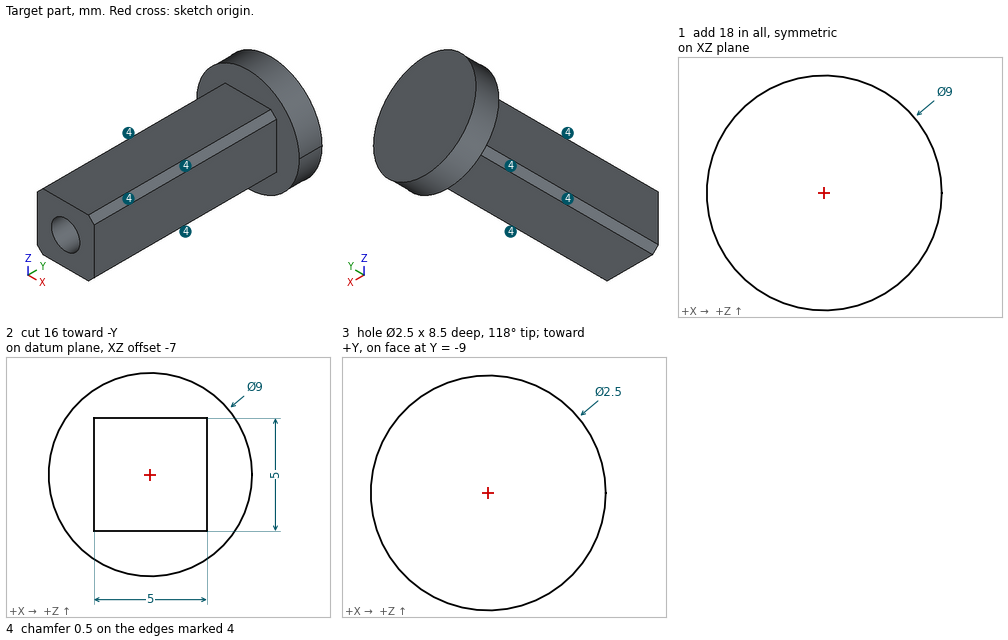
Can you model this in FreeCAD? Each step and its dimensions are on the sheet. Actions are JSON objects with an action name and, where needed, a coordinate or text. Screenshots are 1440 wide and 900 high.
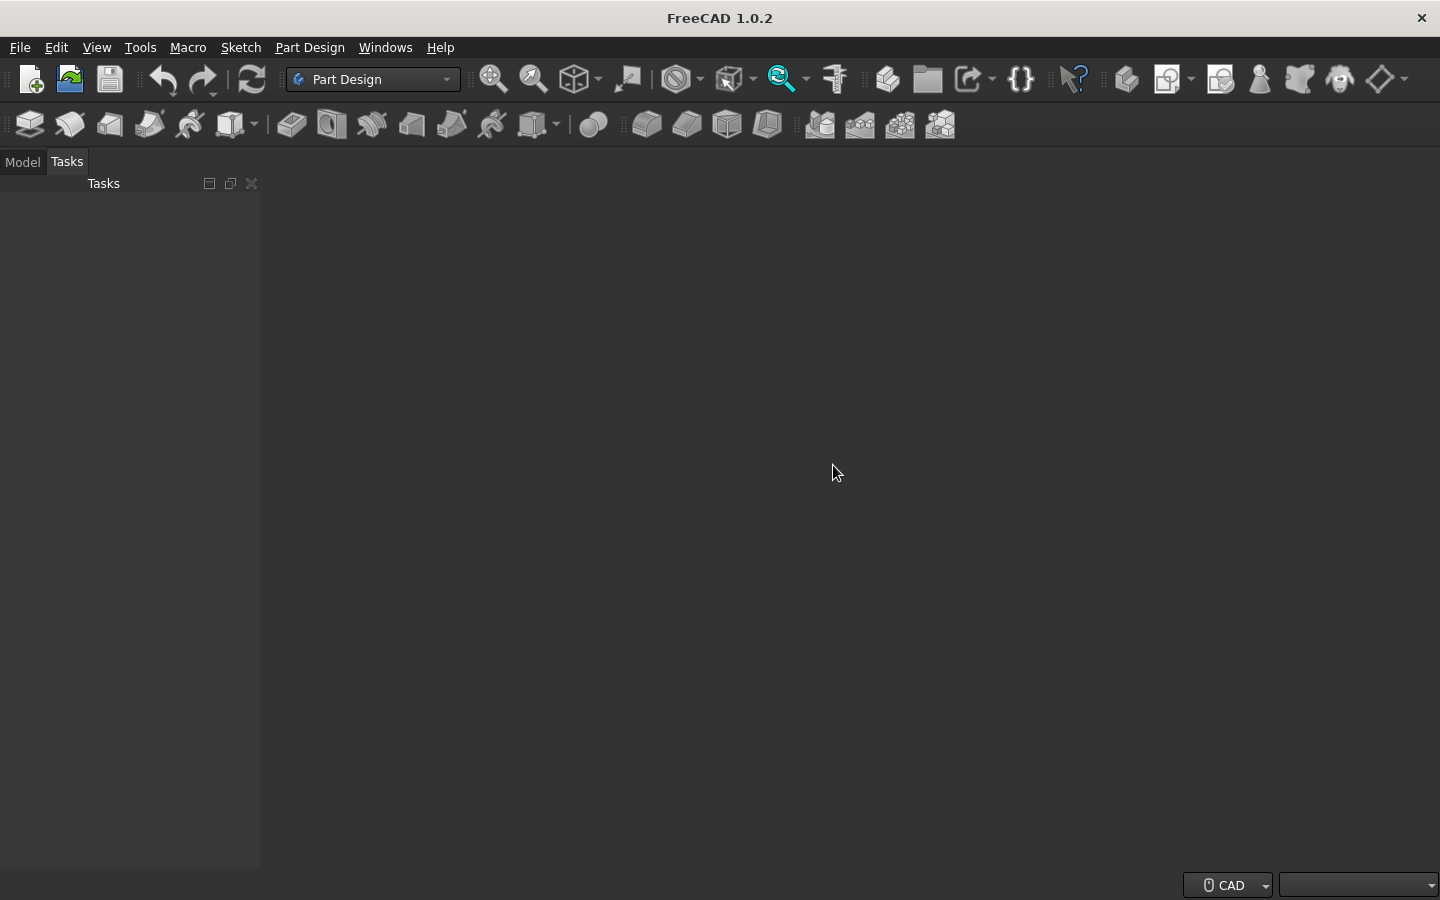
{"action": "left_click", "coordinate": [30, 80]}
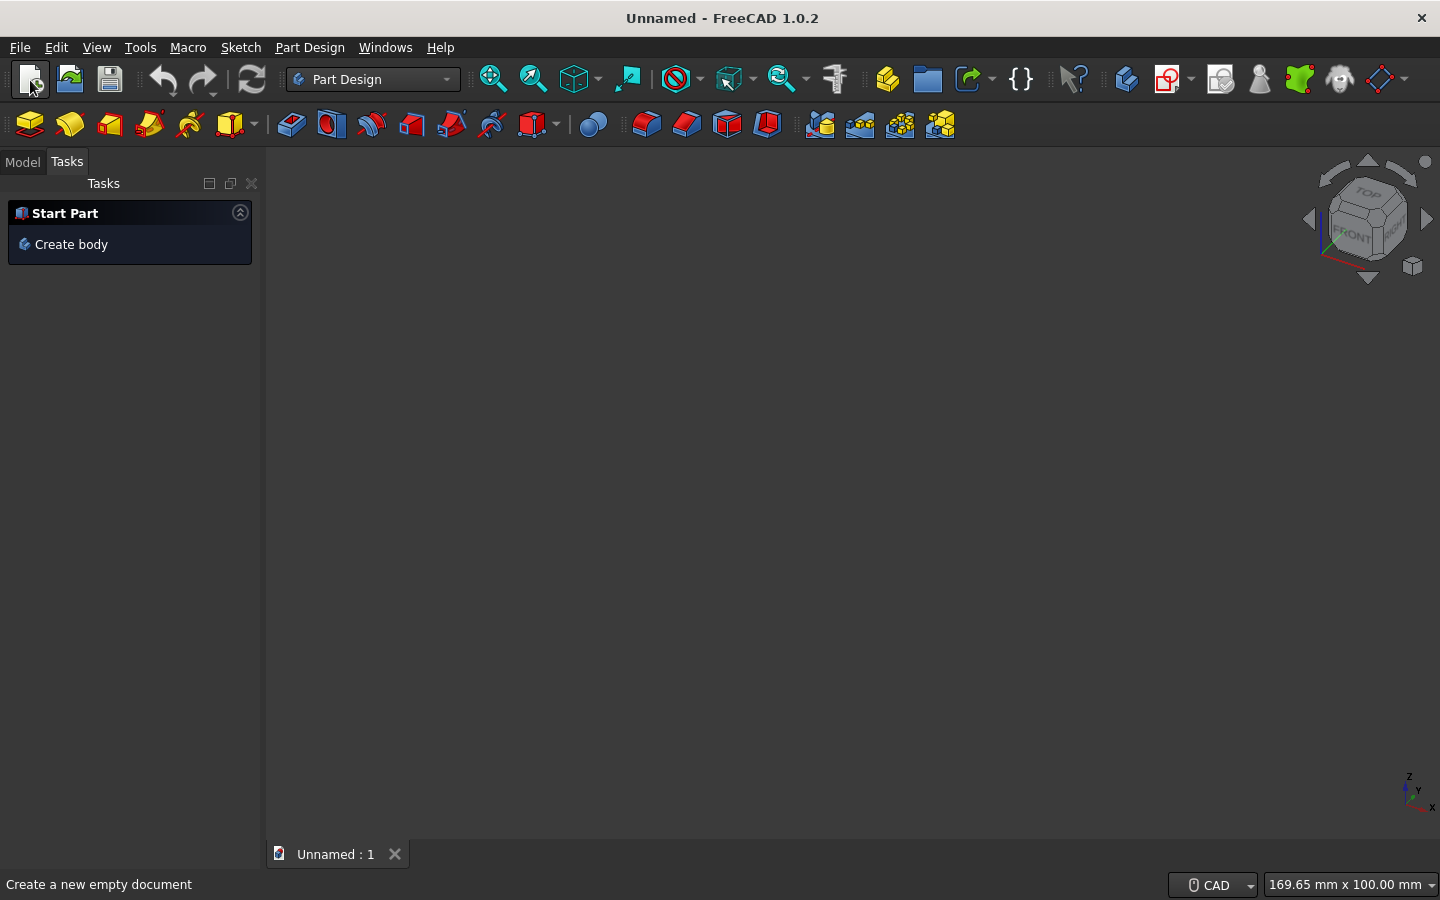
{"action": "left_click", "coordinate": [1168, 80]}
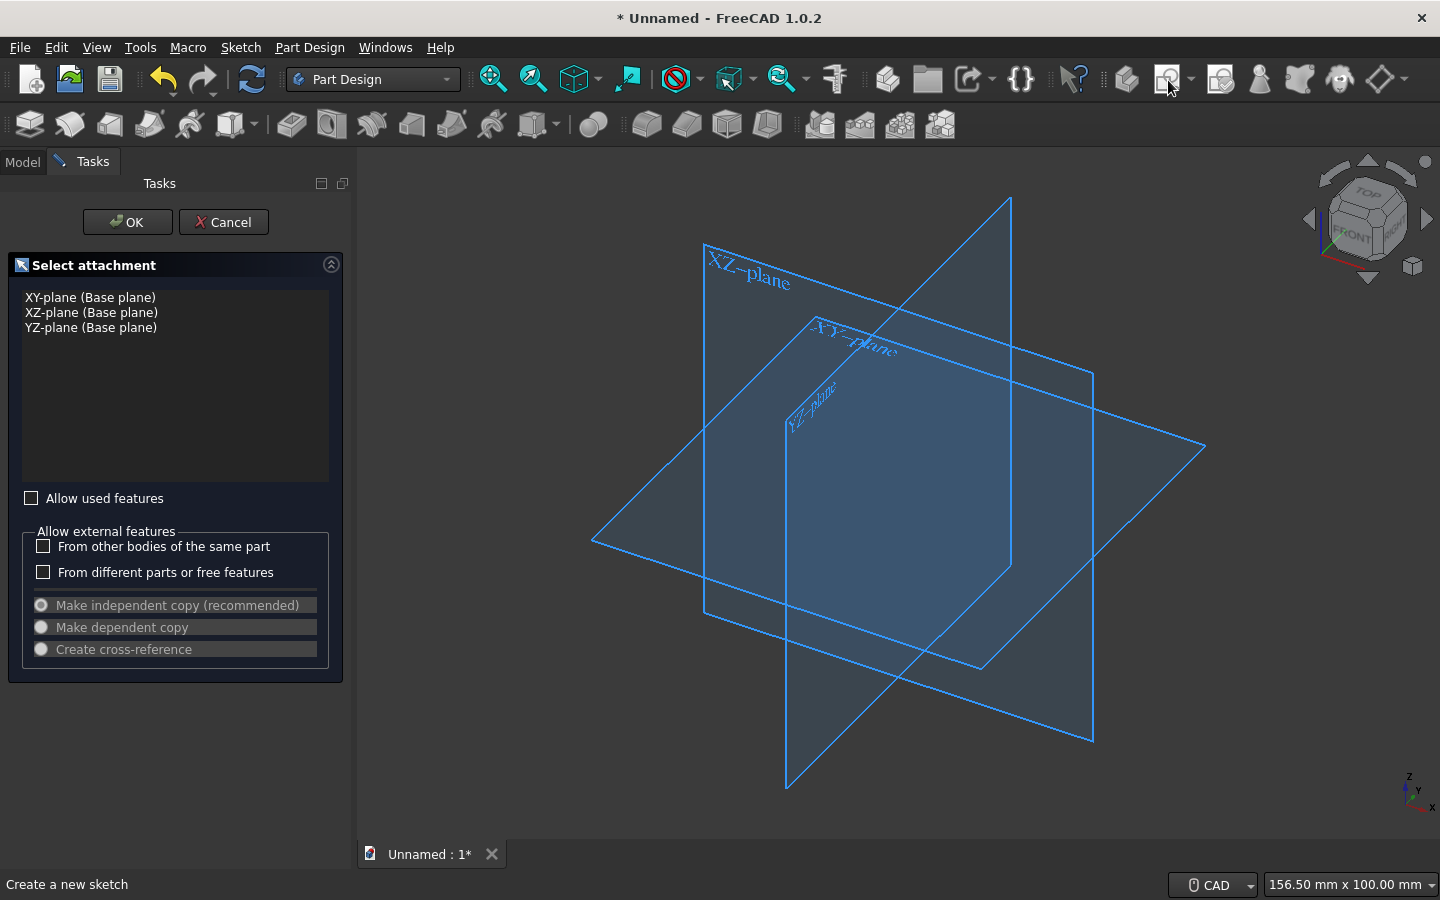
{"action": "left_click", "coordinate": [82, 312]}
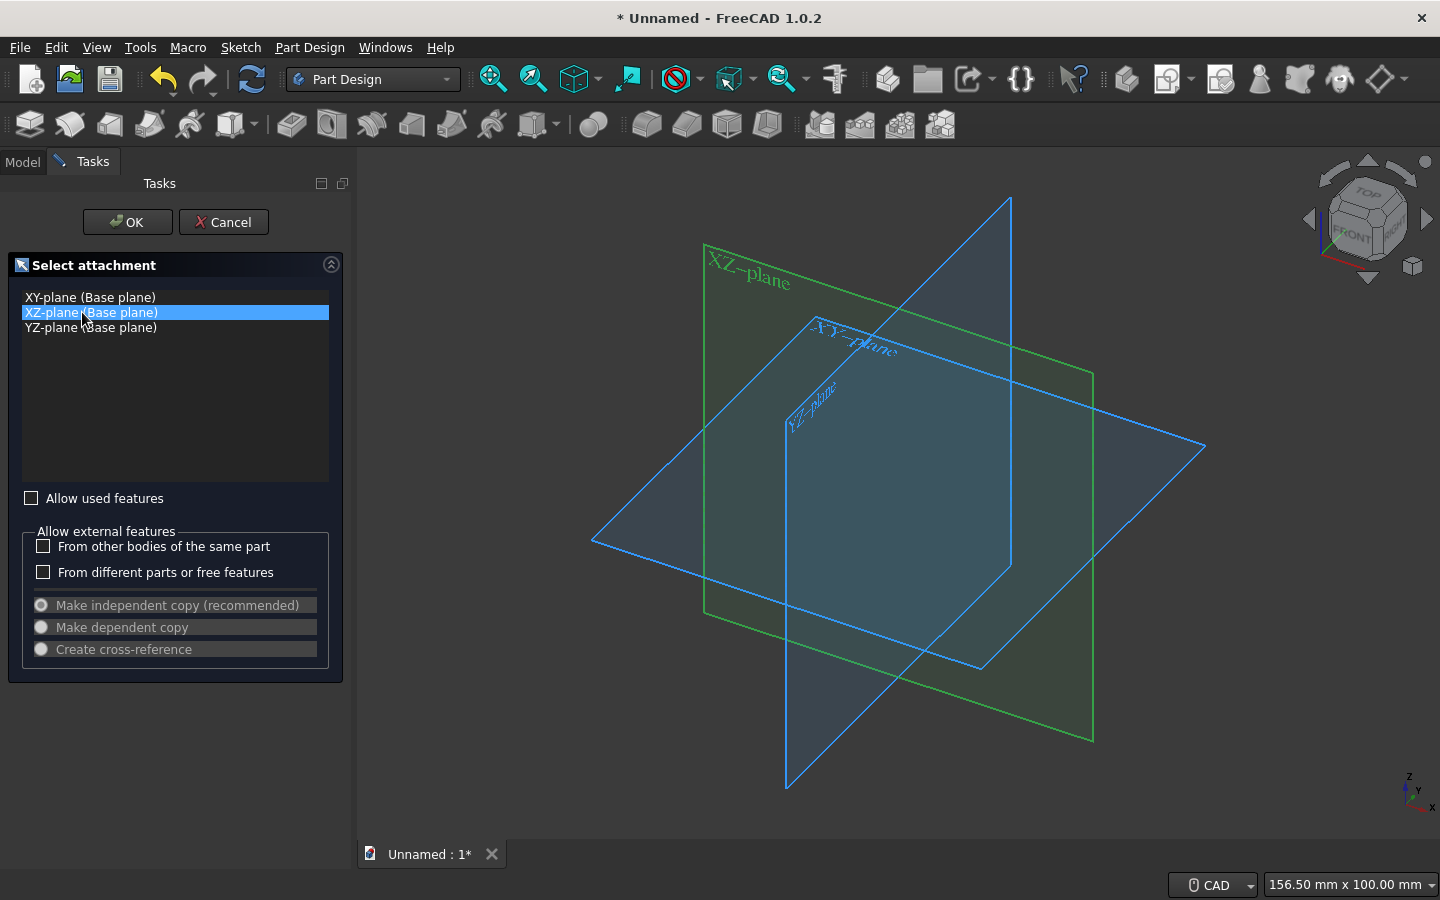
{"action": "left_click", "coordinate": [128, 222]}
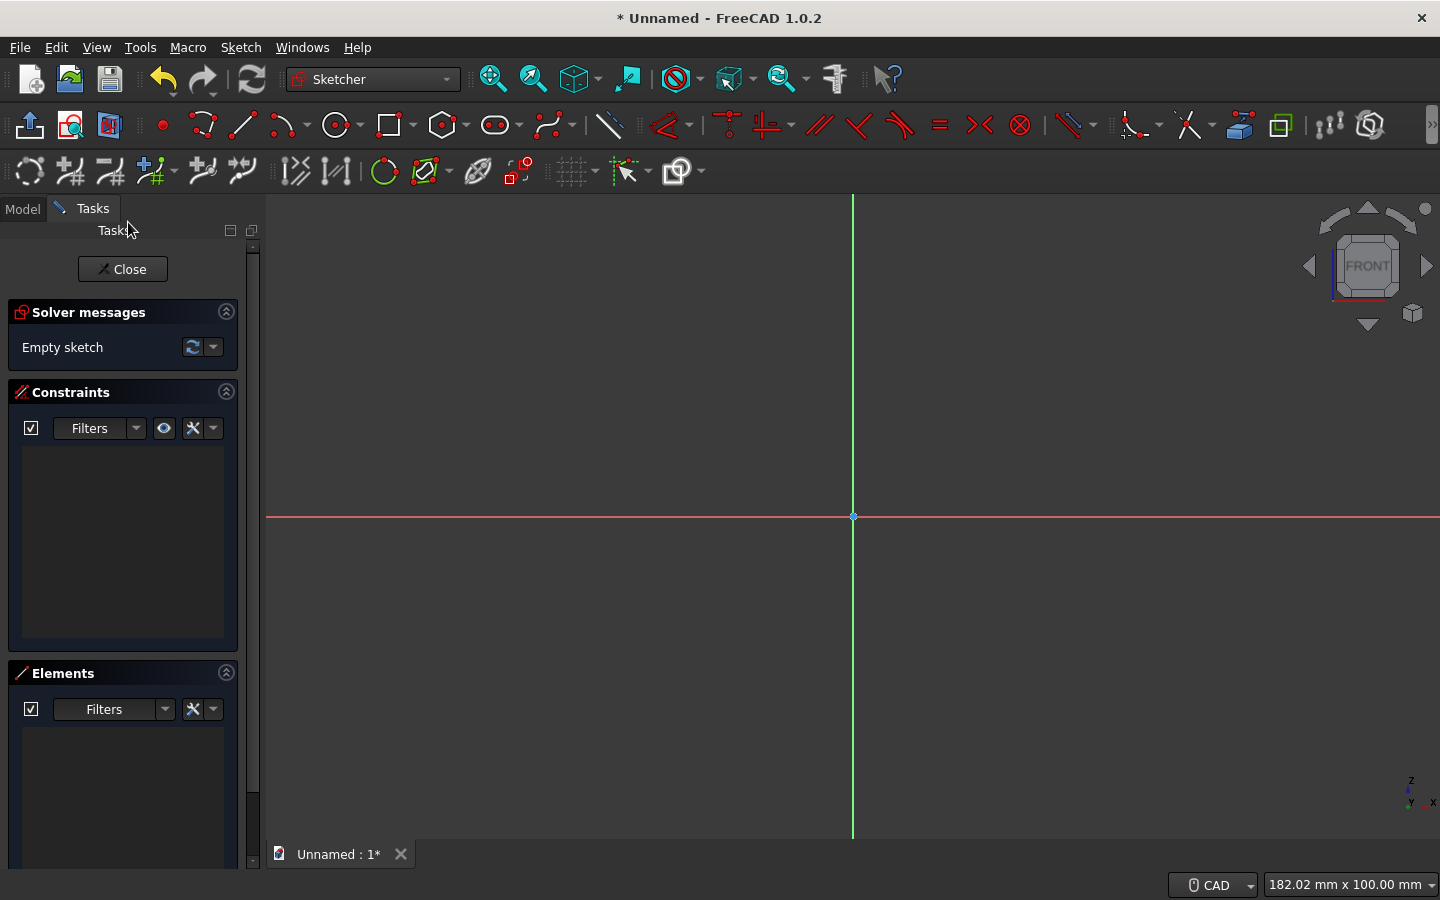
{"action": "scroll", "coordinate": [864, 516], "scroll_direction": "up", "scroll_amount": 10}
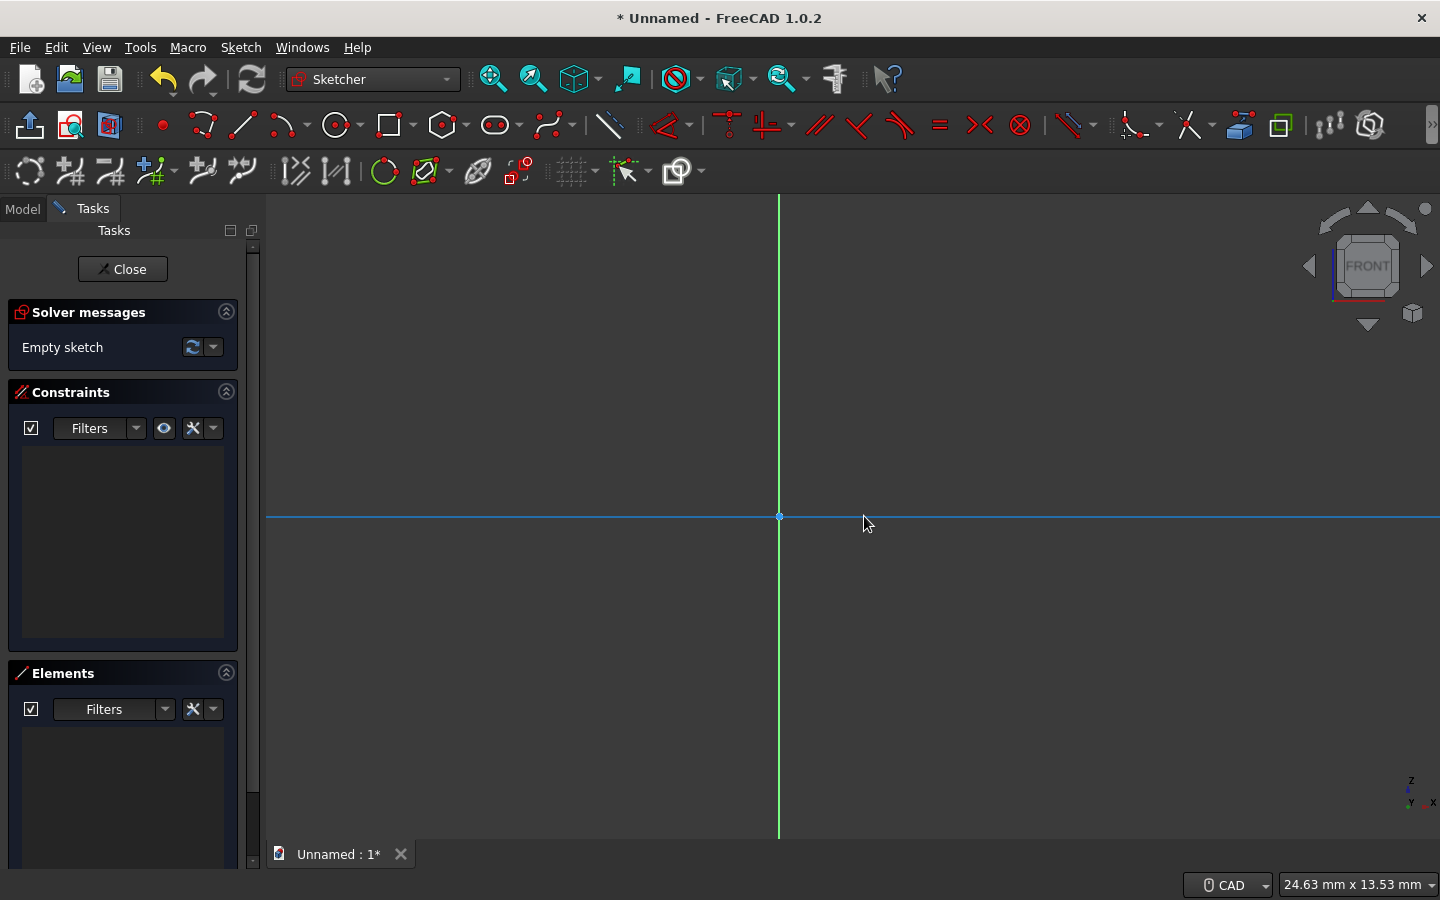
{"action": "left_click", "coordinate": [336, 126]}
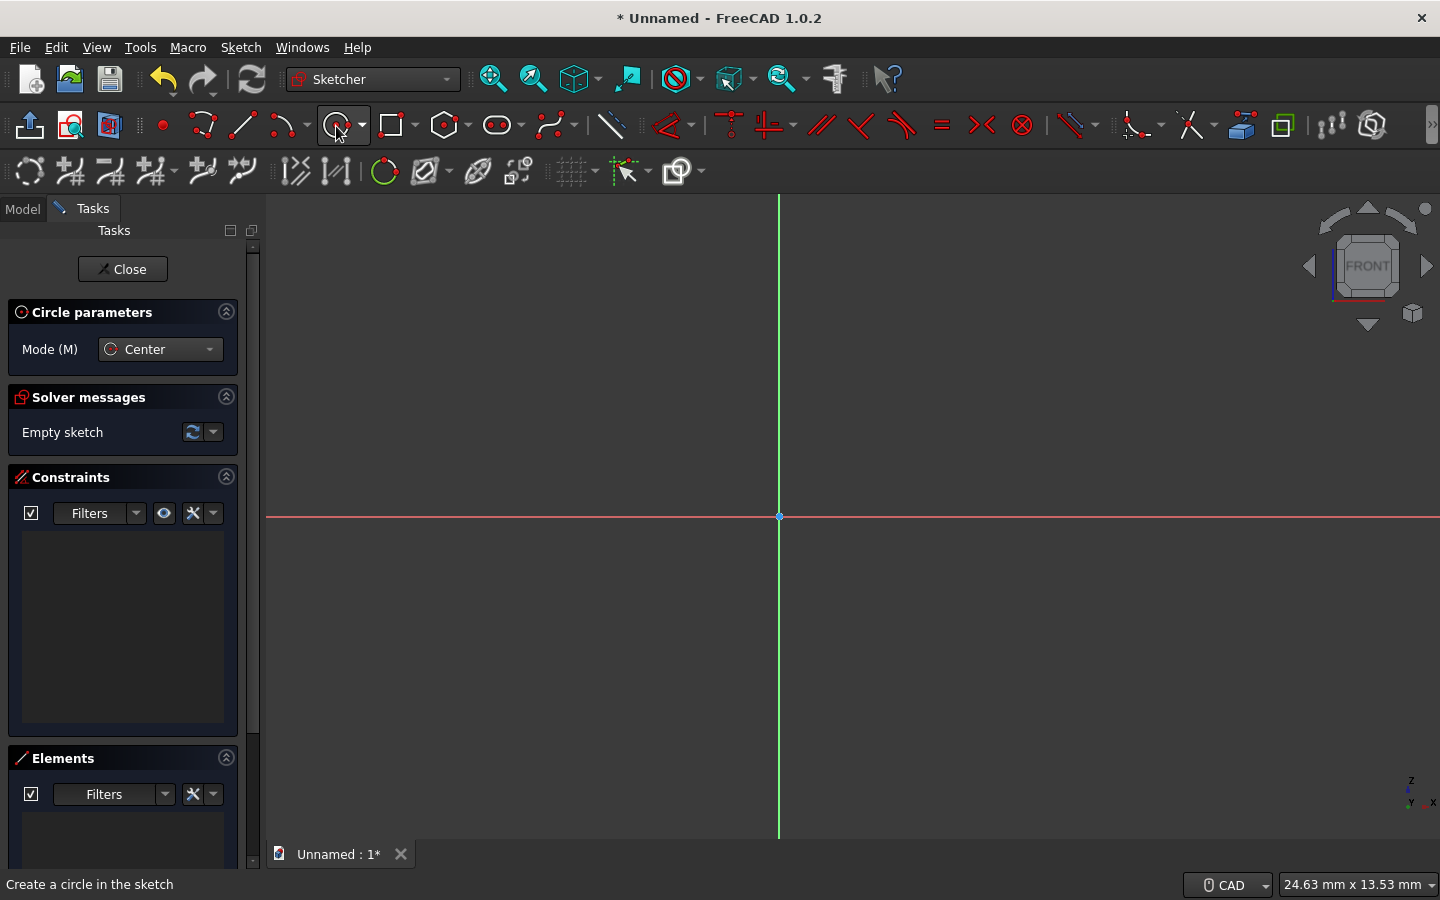
{"action": "left_click", "coordinate": [779, 516]}
{"action": "mouse_move", "coordinate": [931, 365]}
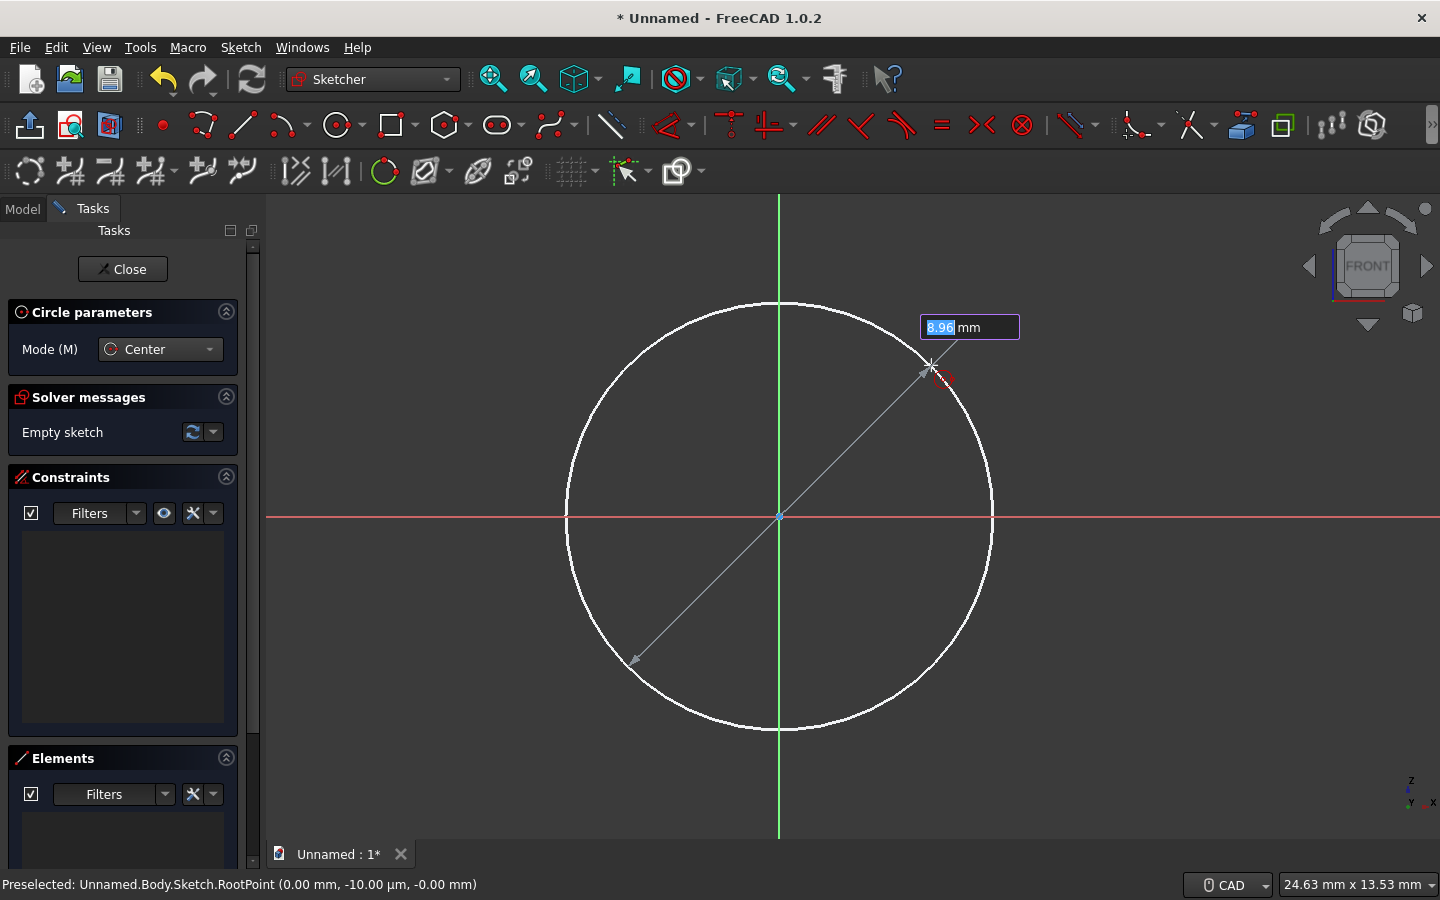
{"action": "type", "text": "9"}
{"action": "key", "text": "Return"}
{"action": "key", "text": "Escape"}